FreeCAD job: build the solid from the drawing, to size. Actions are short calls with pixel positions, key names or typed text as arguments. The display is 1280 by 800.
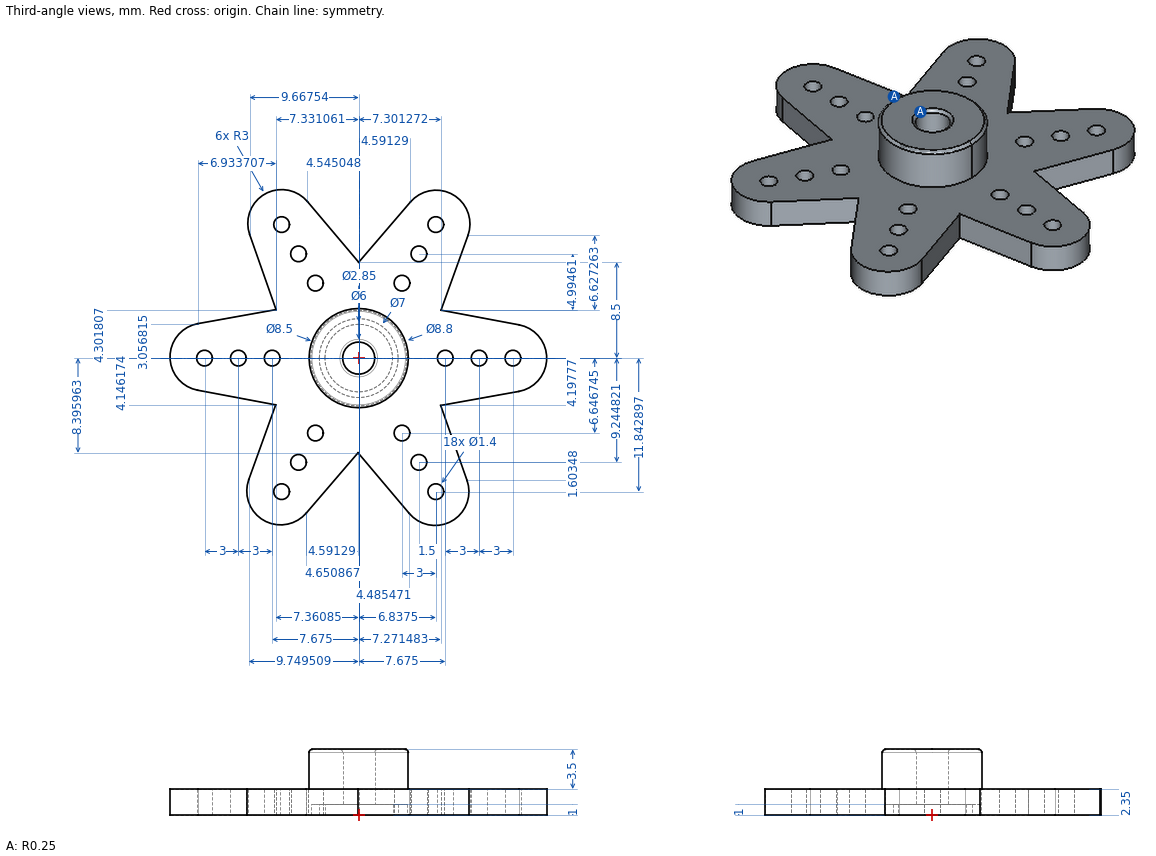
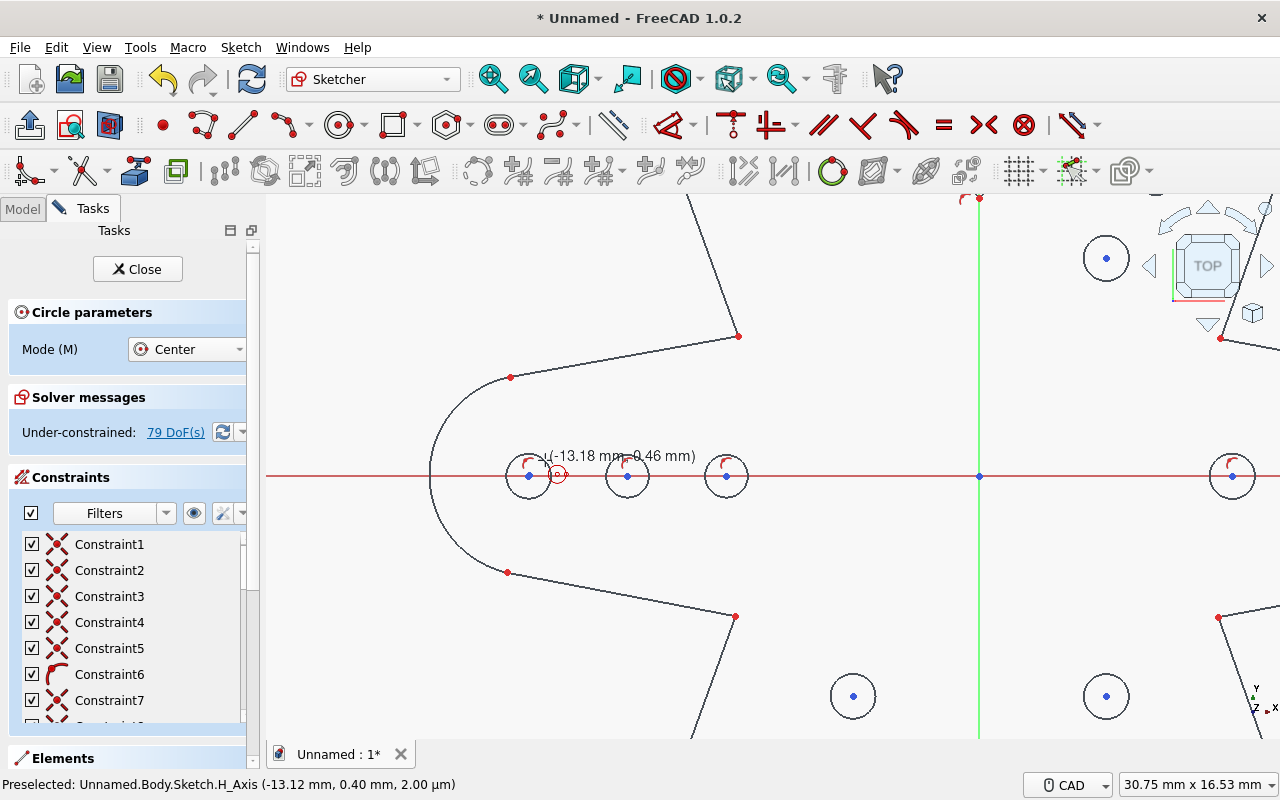
click(853, 257)
click(869, 241)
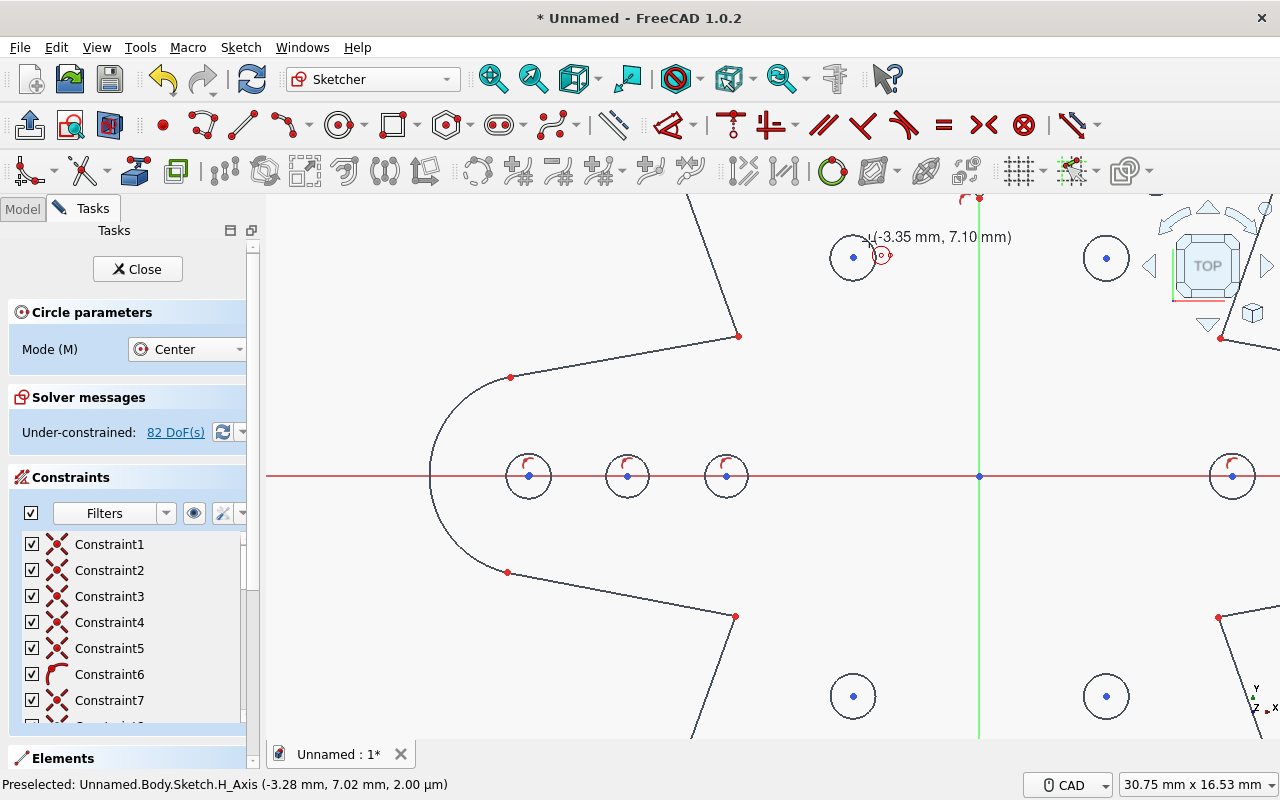
scroll(545, 462, down, 5)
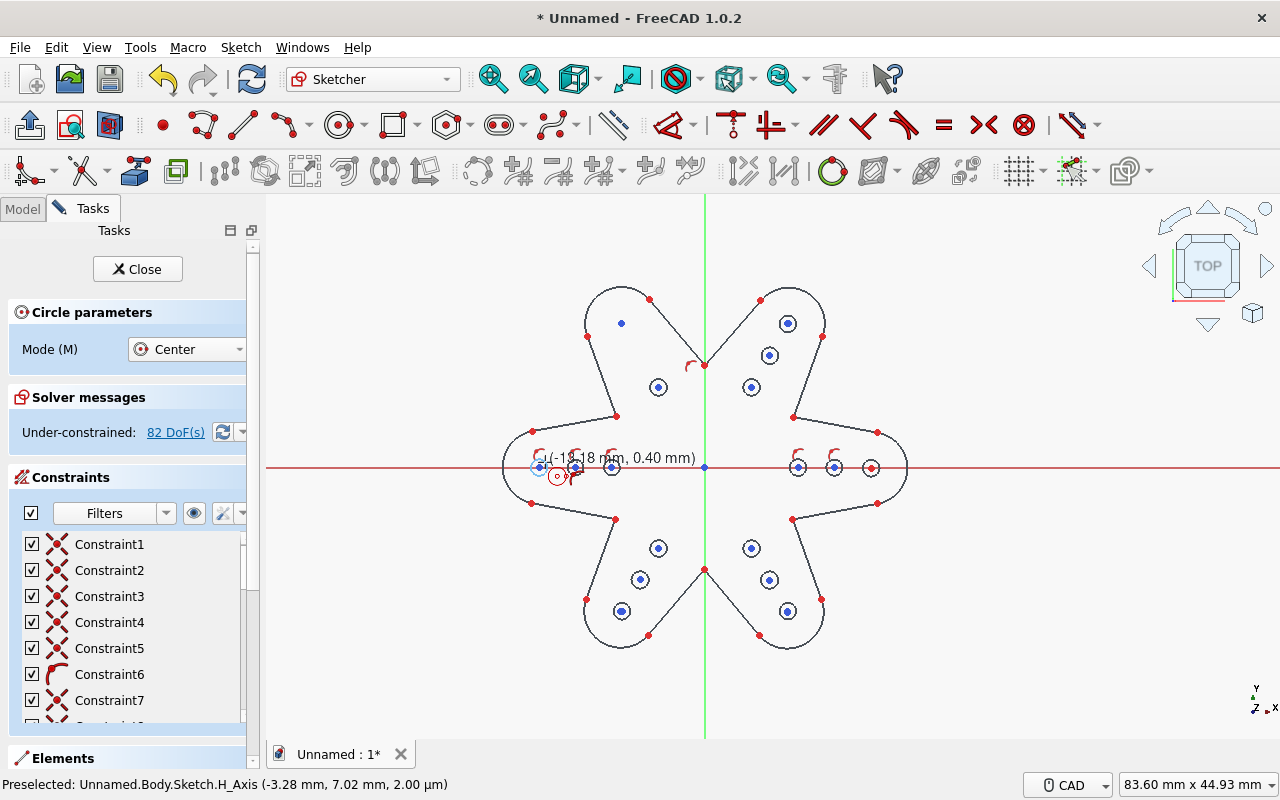
scroll(640, 355, up, 5)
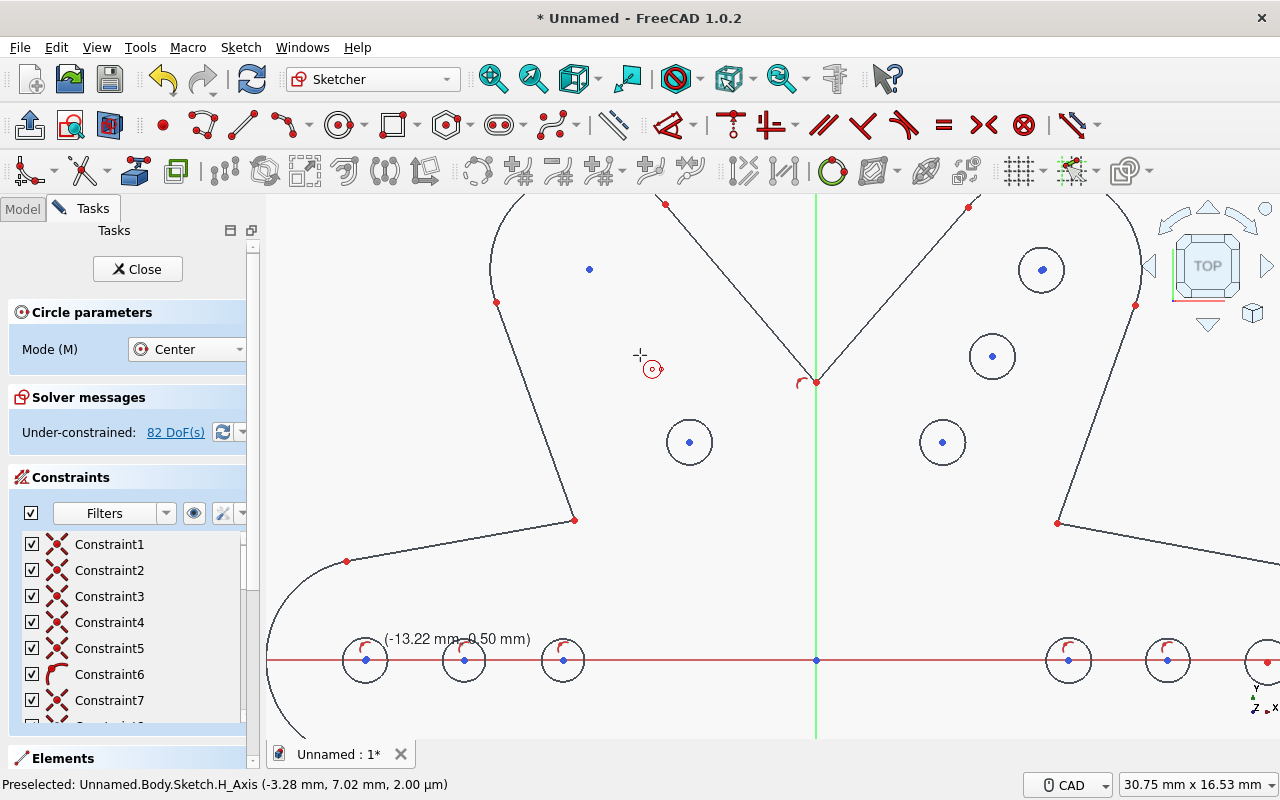
click(640, 356)
click(656, 339)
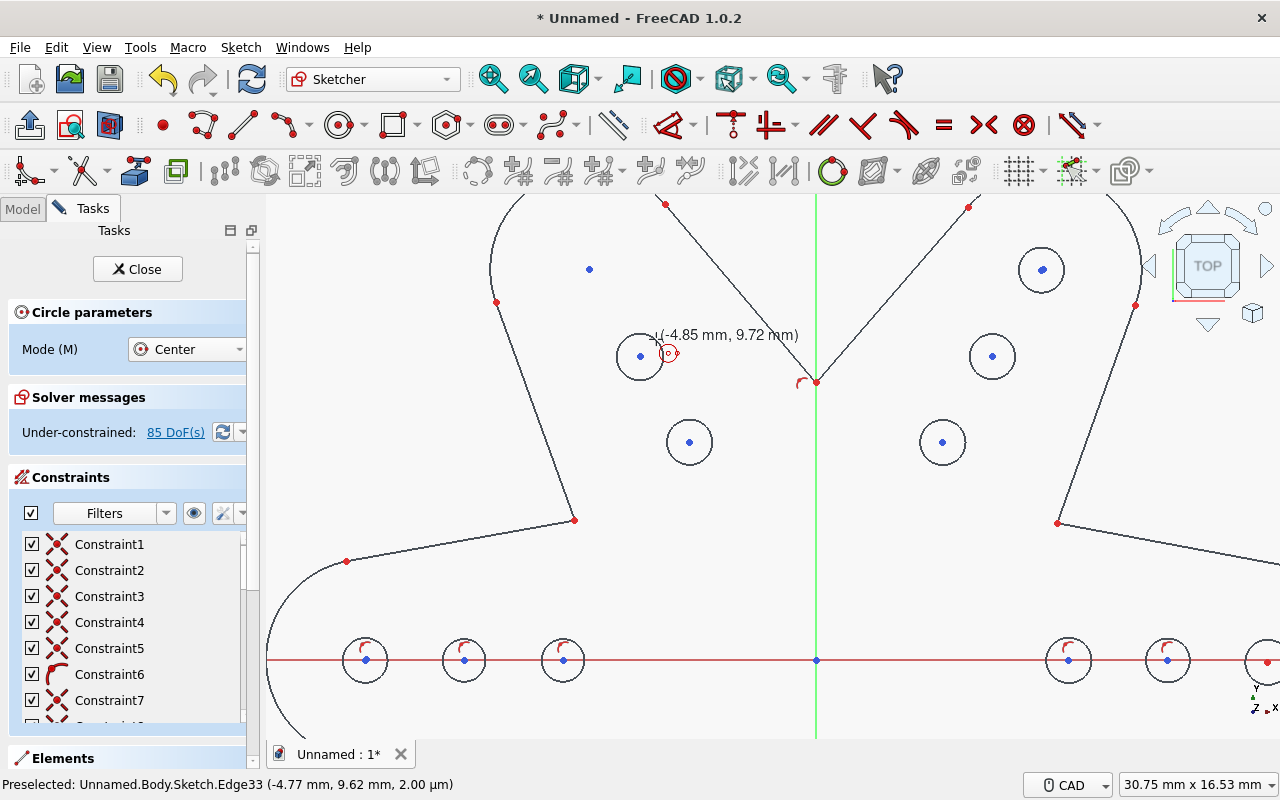
scroll(591, 270, up, 8)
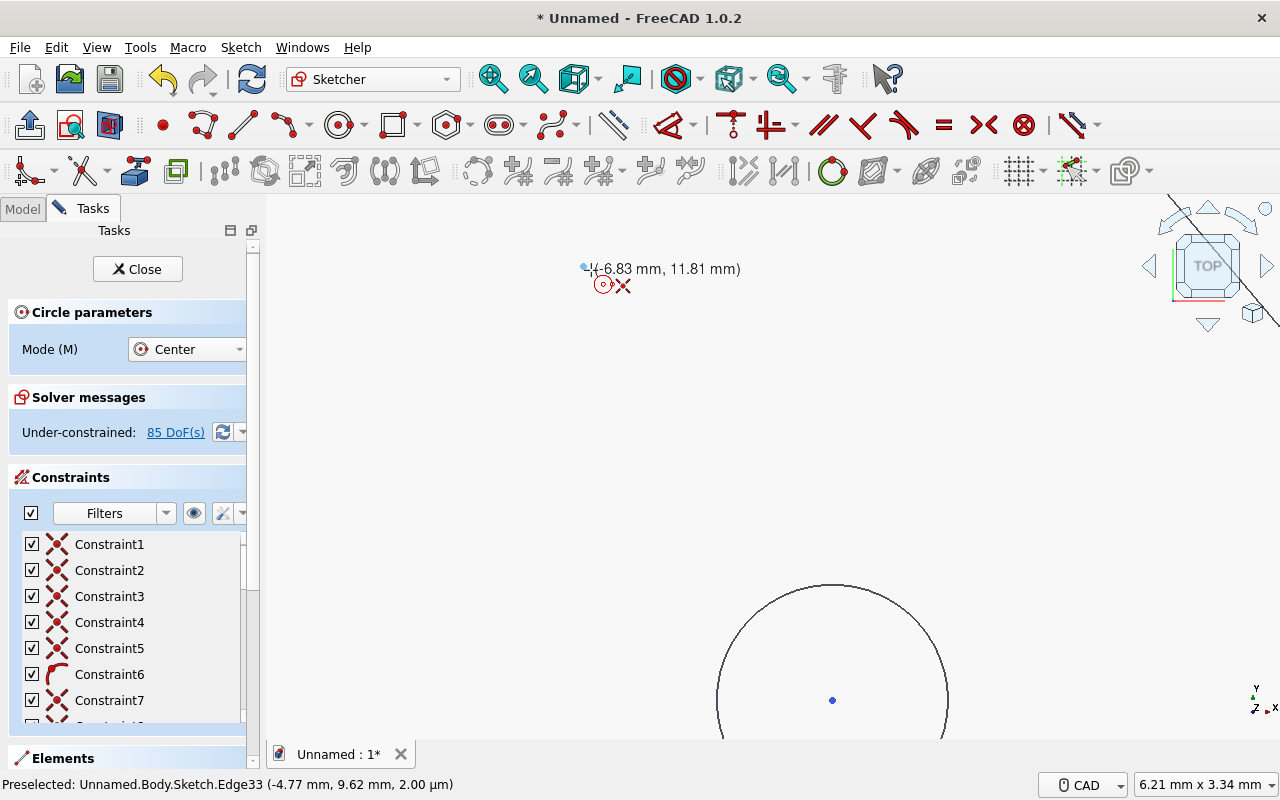
click(588, 269)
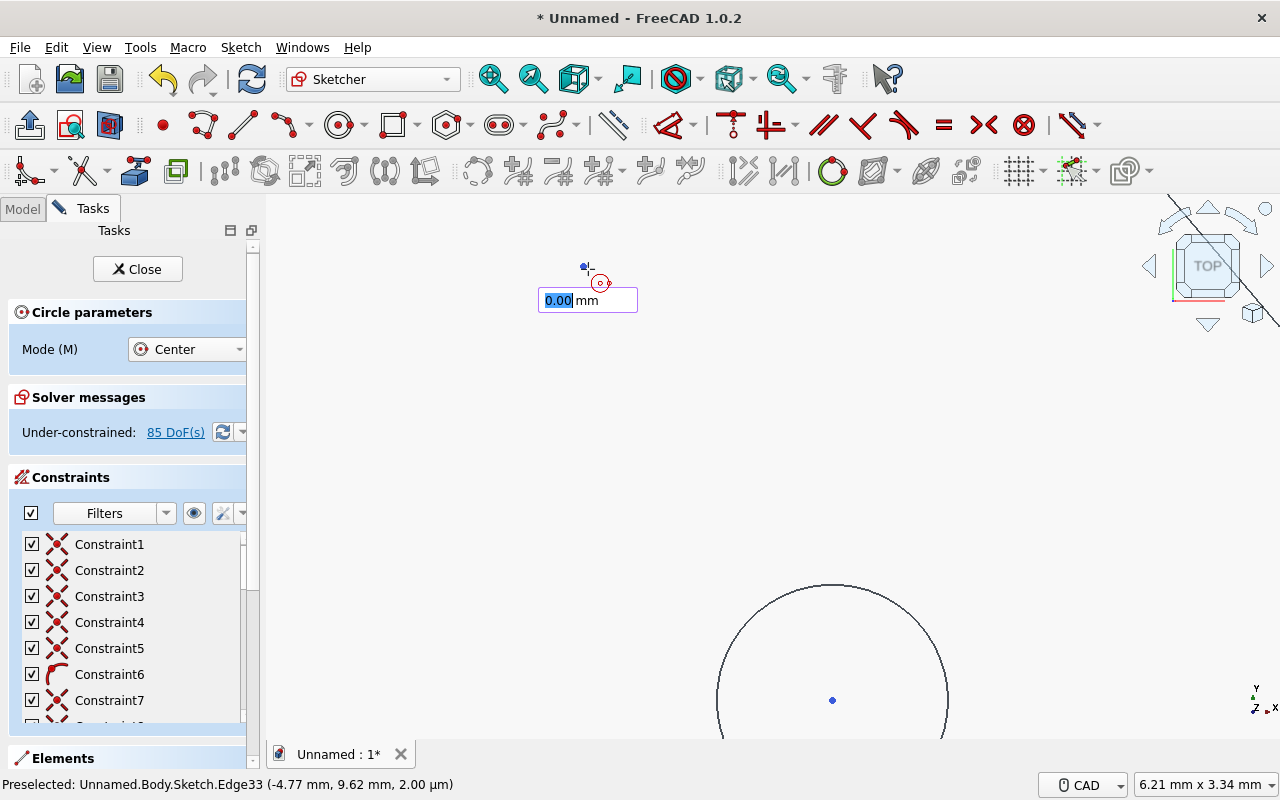
scroll(625, 328, down, 13)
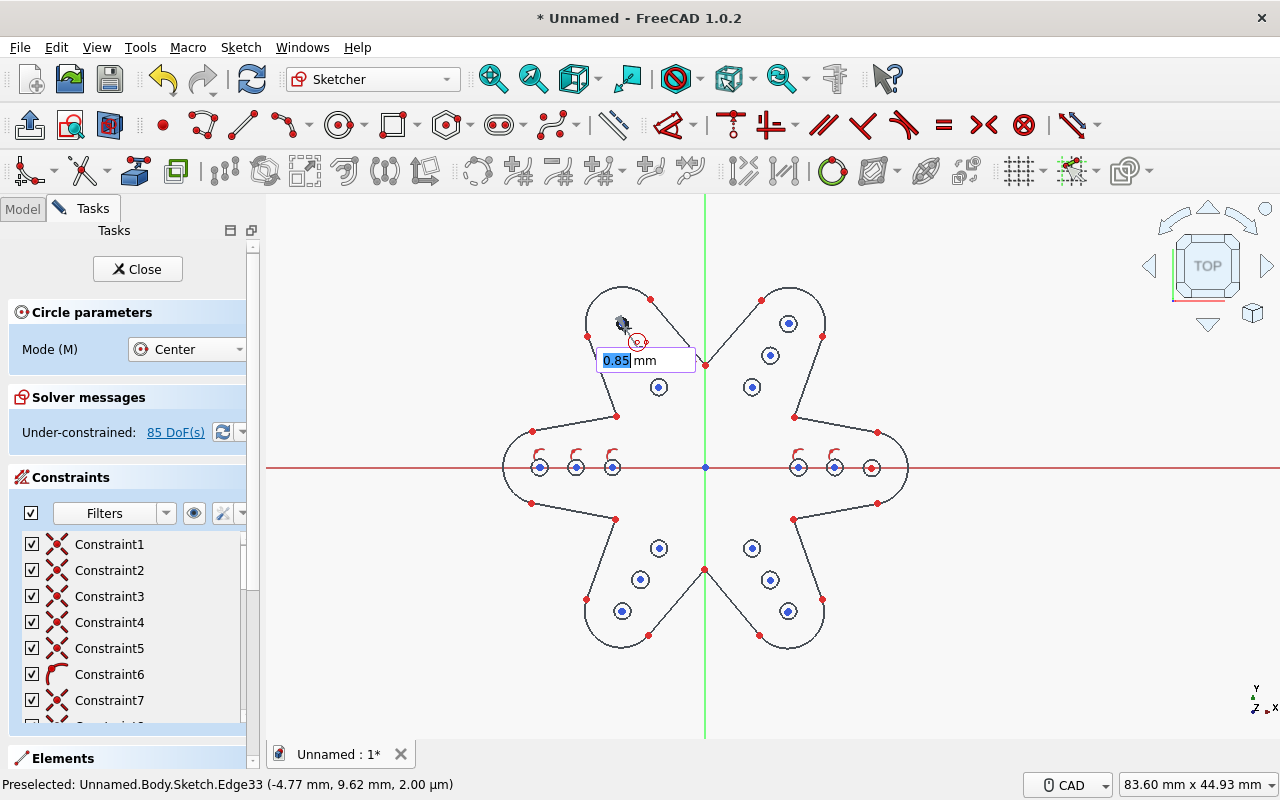
scroll(629, 318, up, 4)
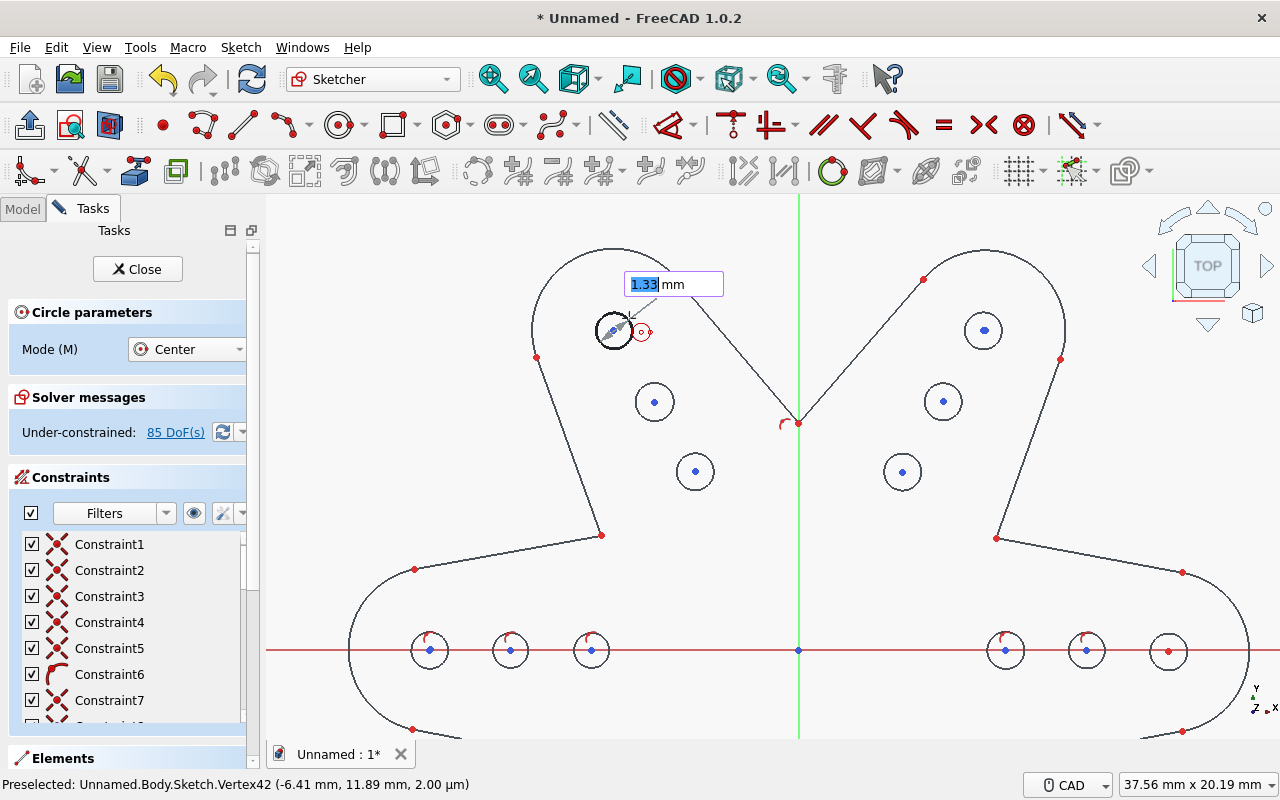
click(628, 317)
key(Escape)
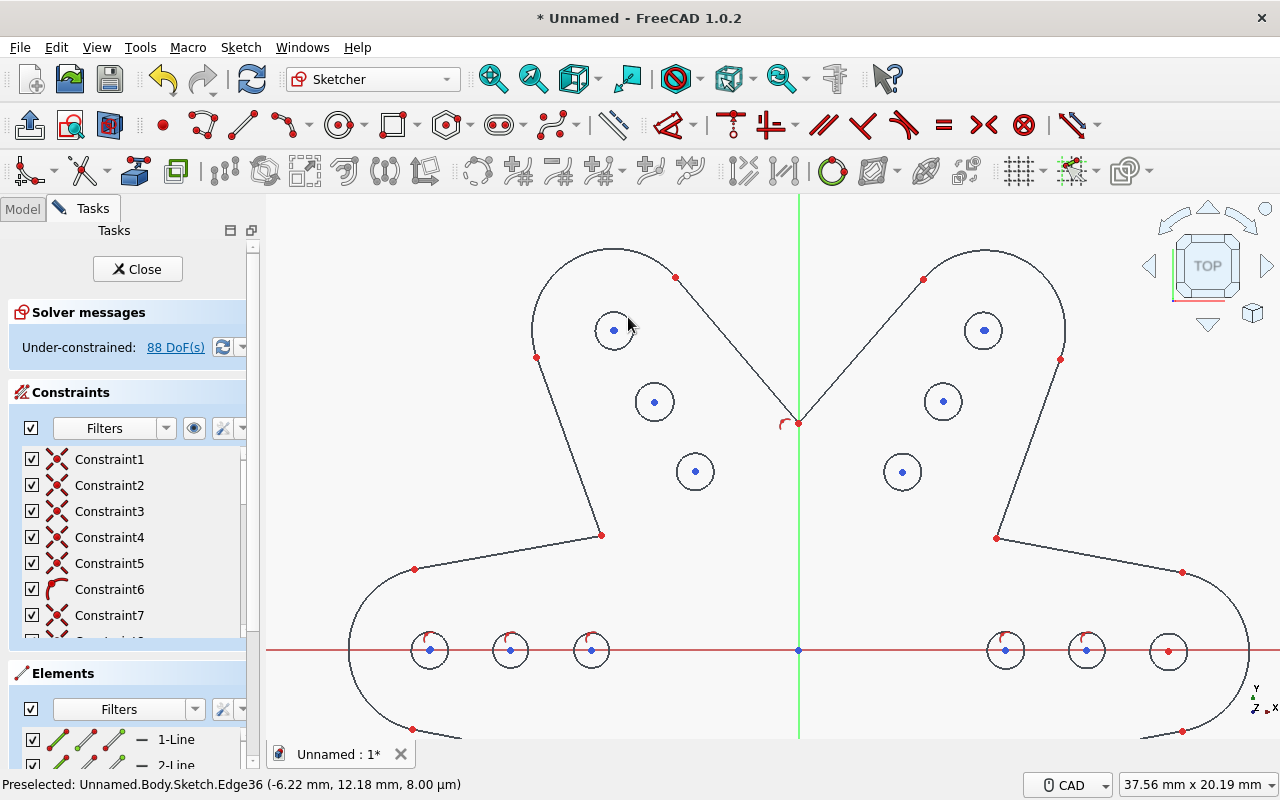
click(556, 411)